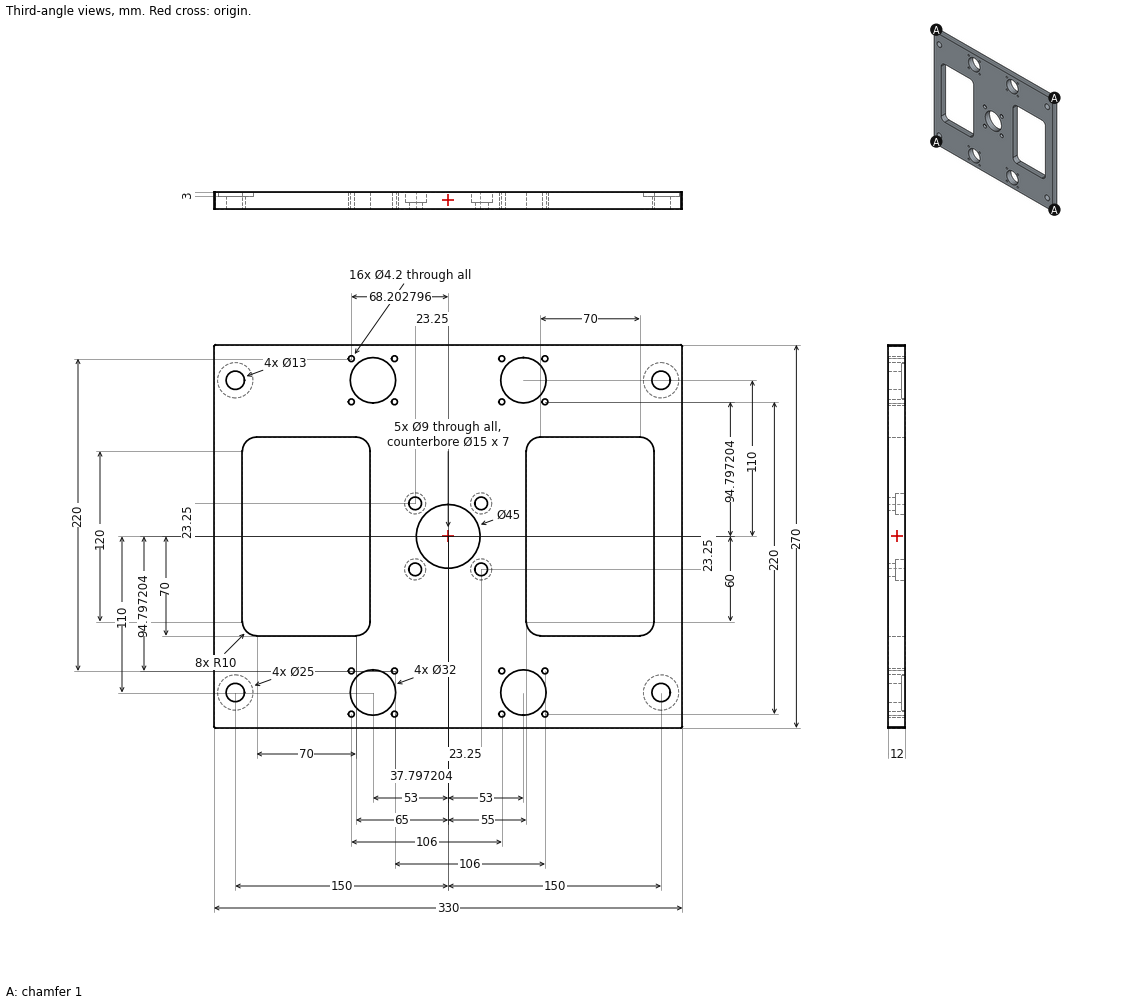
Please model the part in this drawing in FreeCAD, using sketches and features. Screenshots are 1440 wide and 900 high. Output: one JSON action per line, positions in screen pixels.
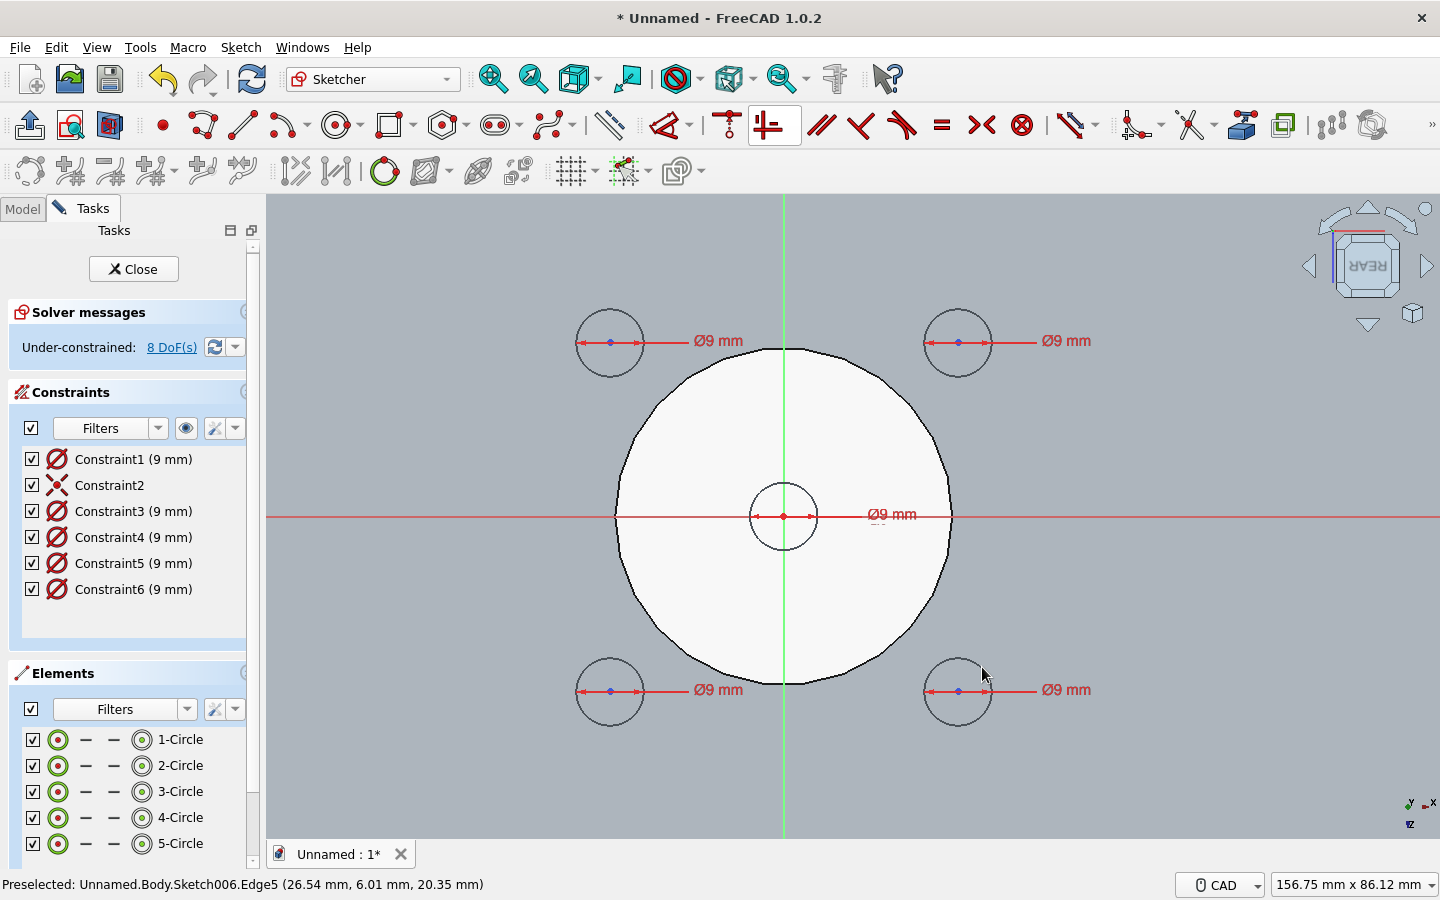
{"action": "left_click", "coordinate": [610, 692]}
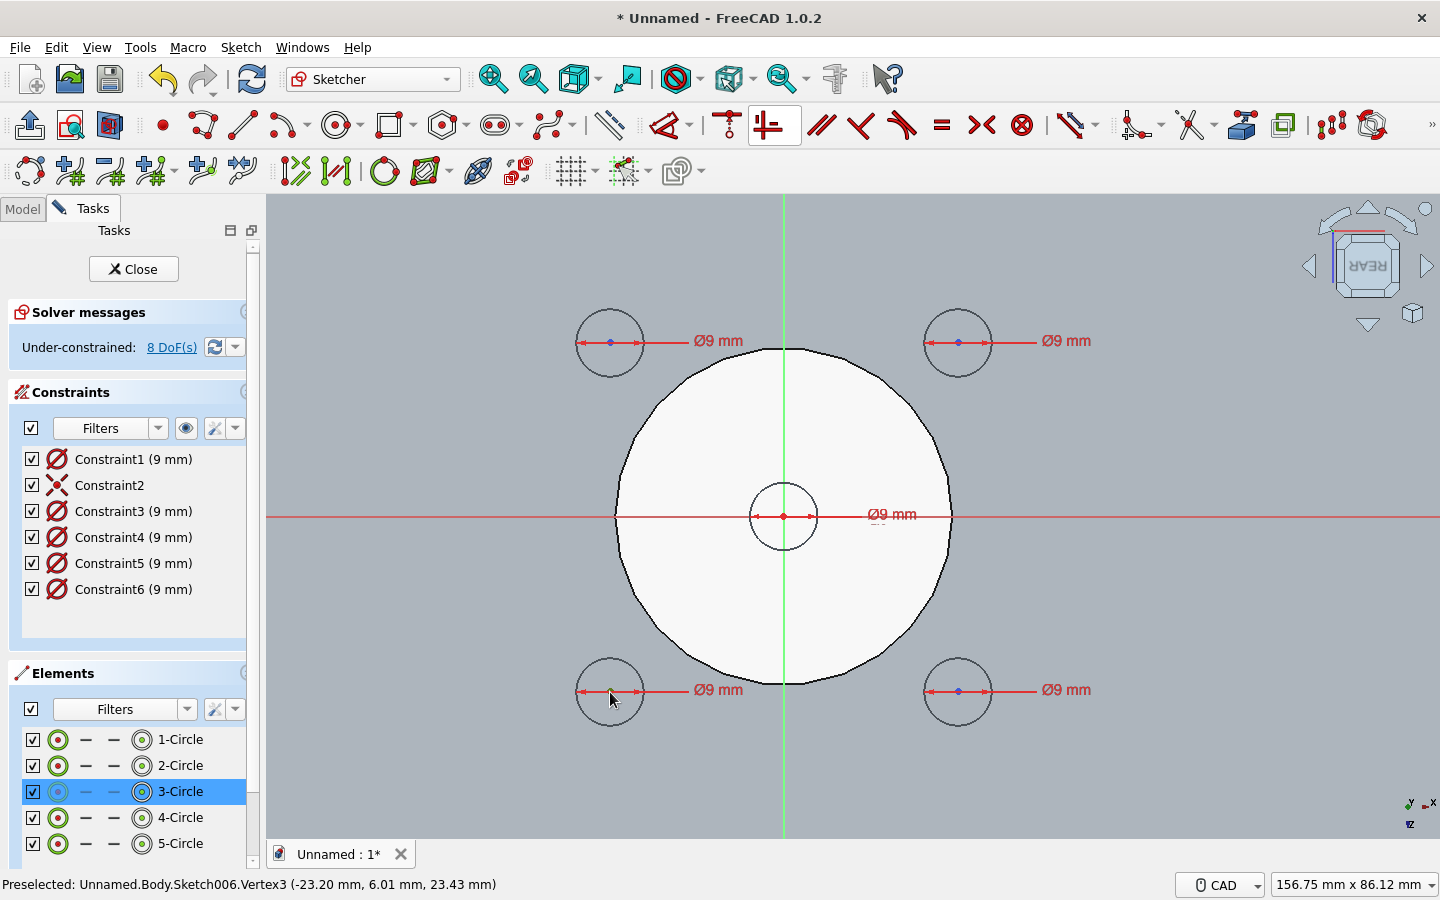
{"action": "left_click", "coordinate": [610, 343]}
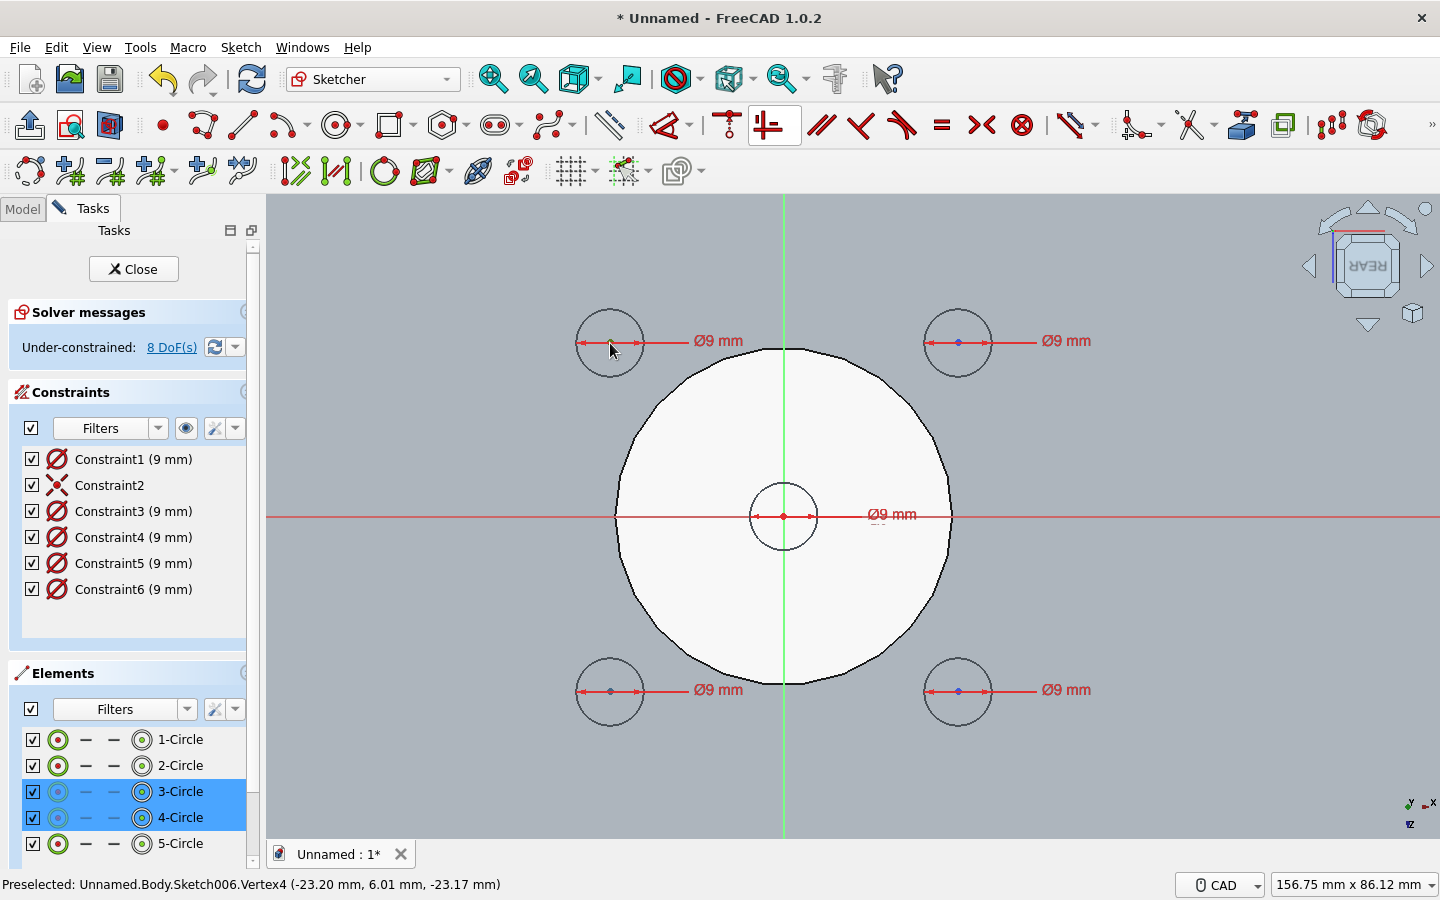
{"action": "key", "text": "v"}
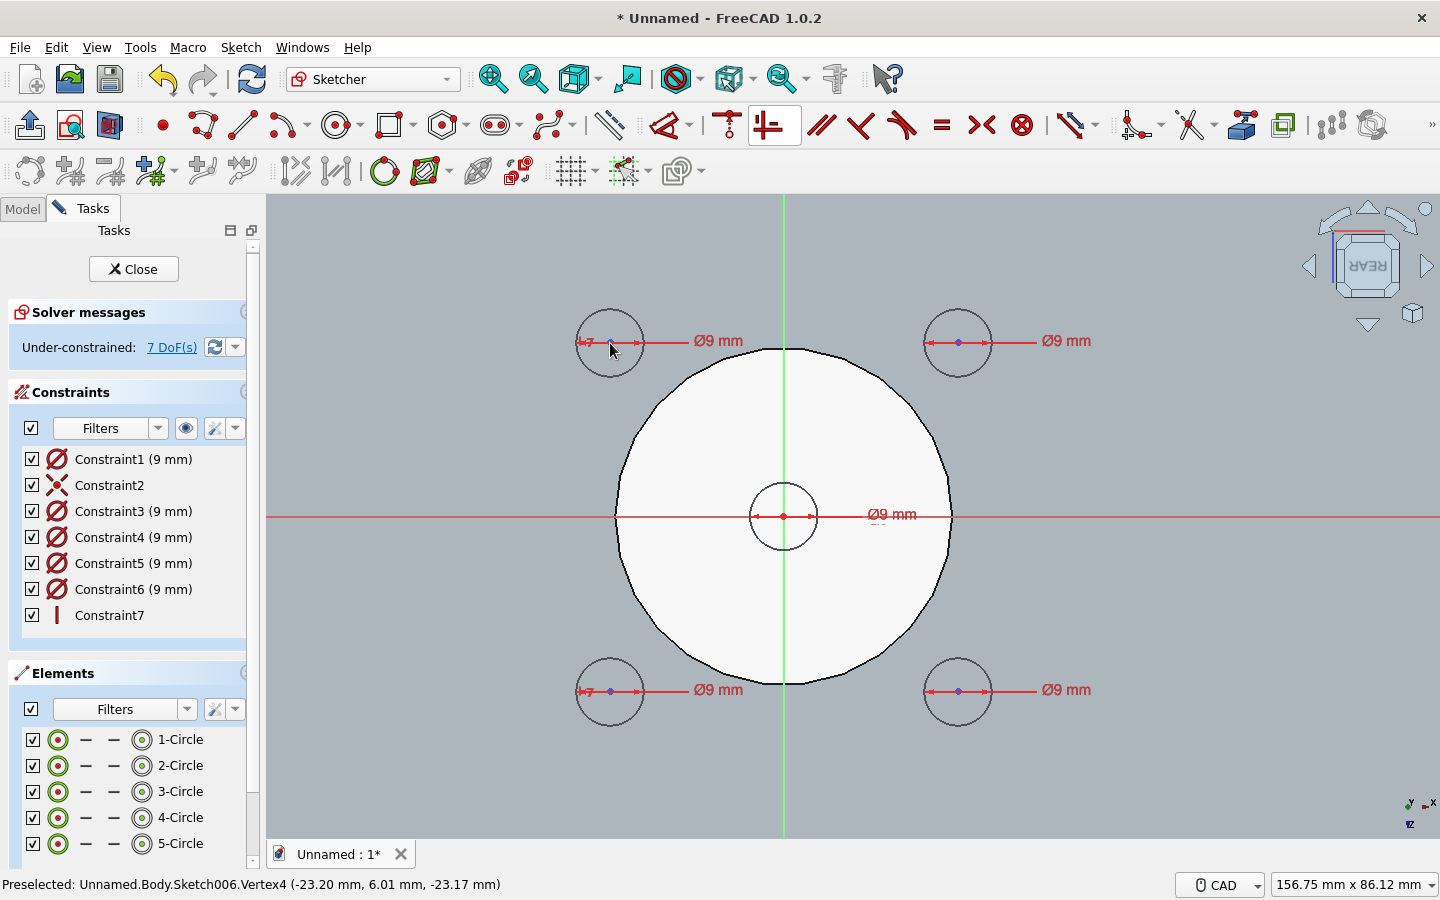
{"action": "left_click", "coordinate": [958, 343]}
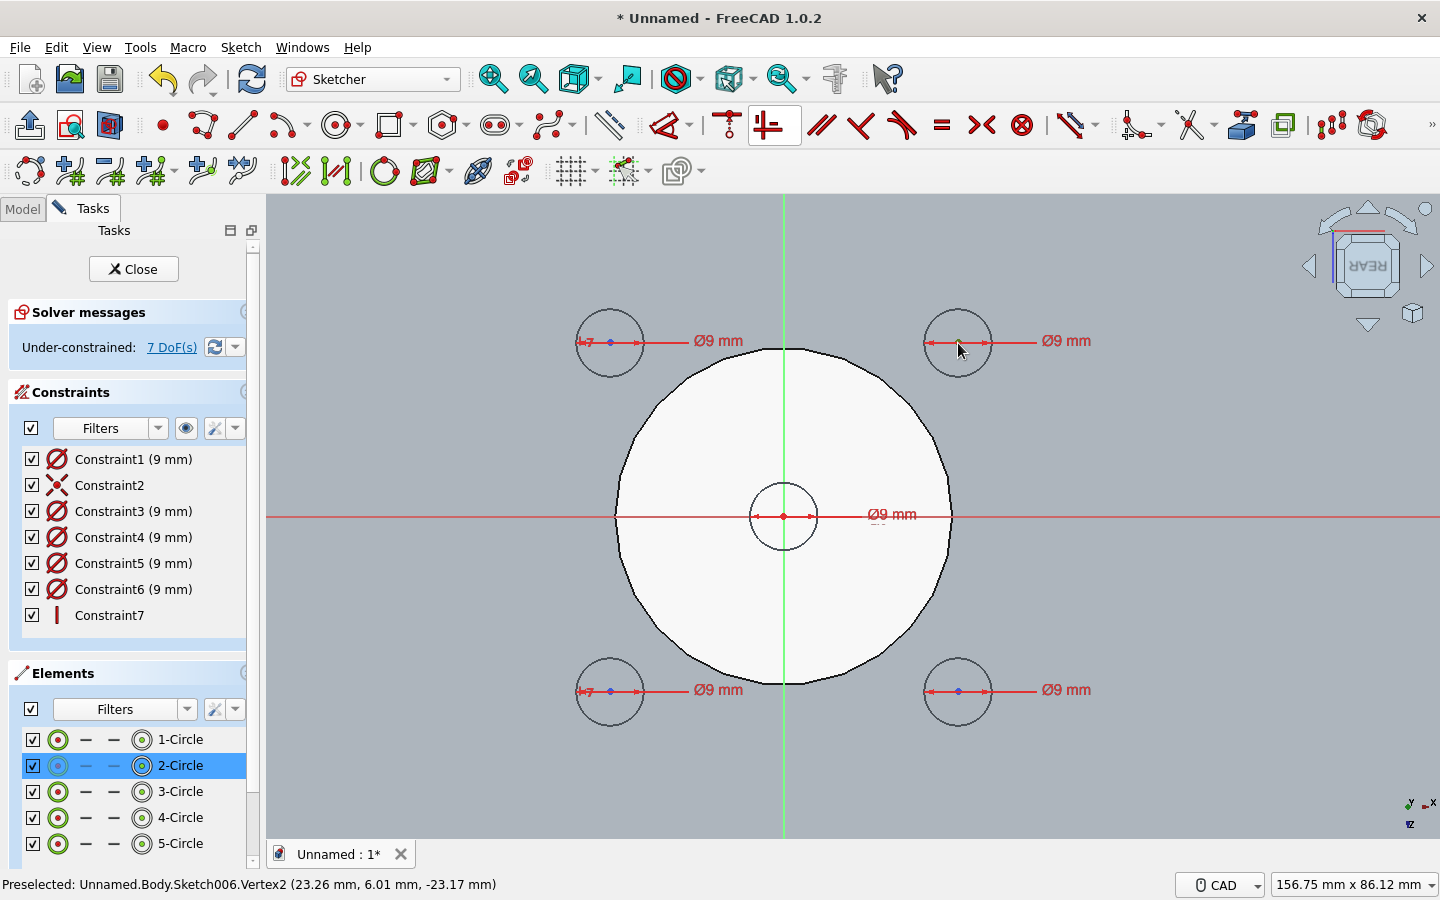
{"action": "left_click", "coordinate": [610, 343]}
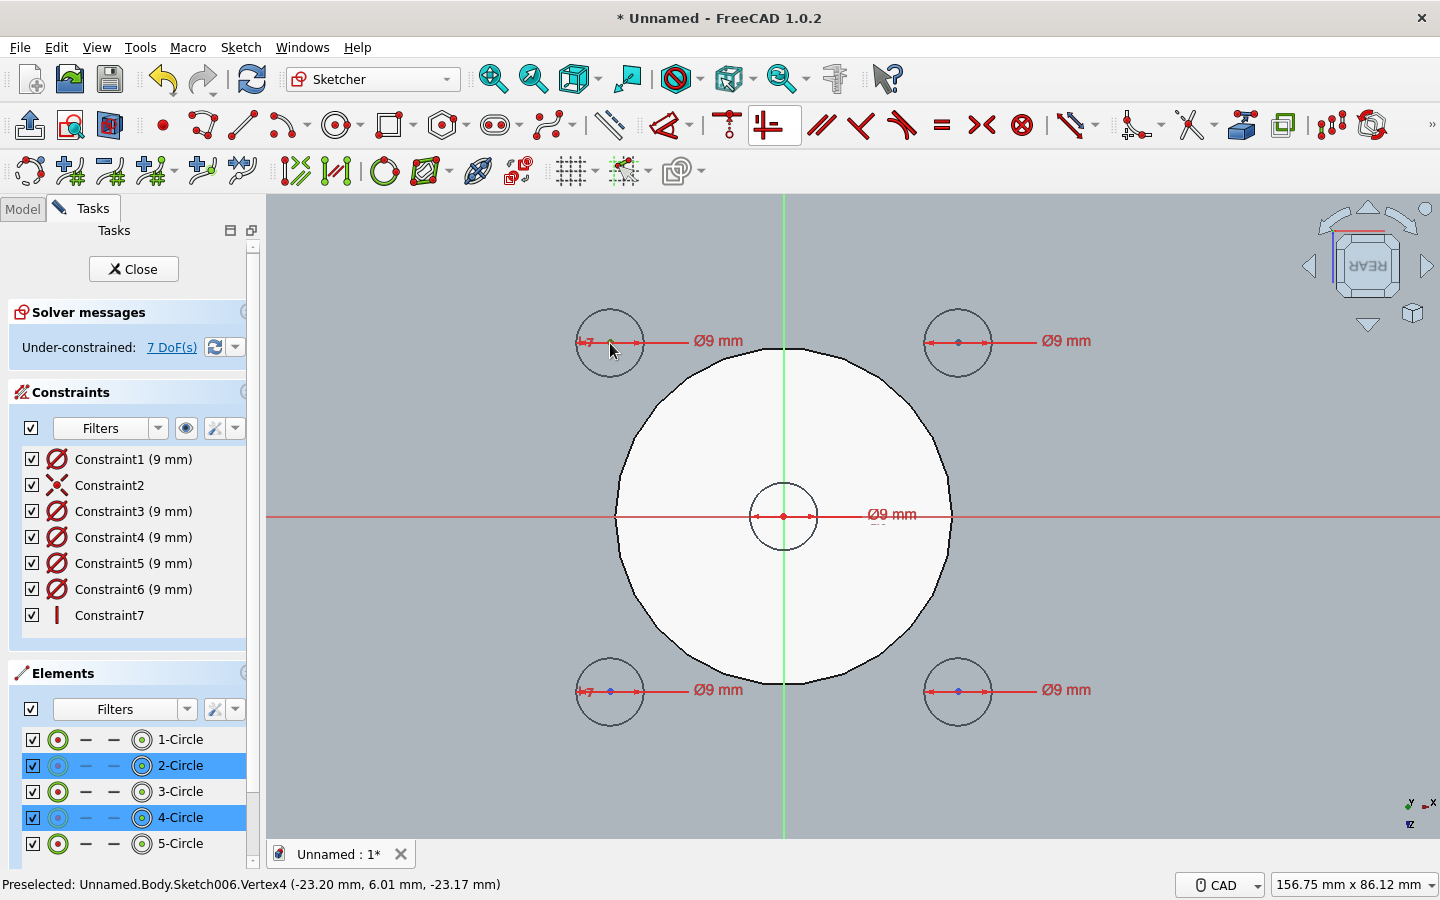
{"action": "left_click", "coordinate": [796, 126]}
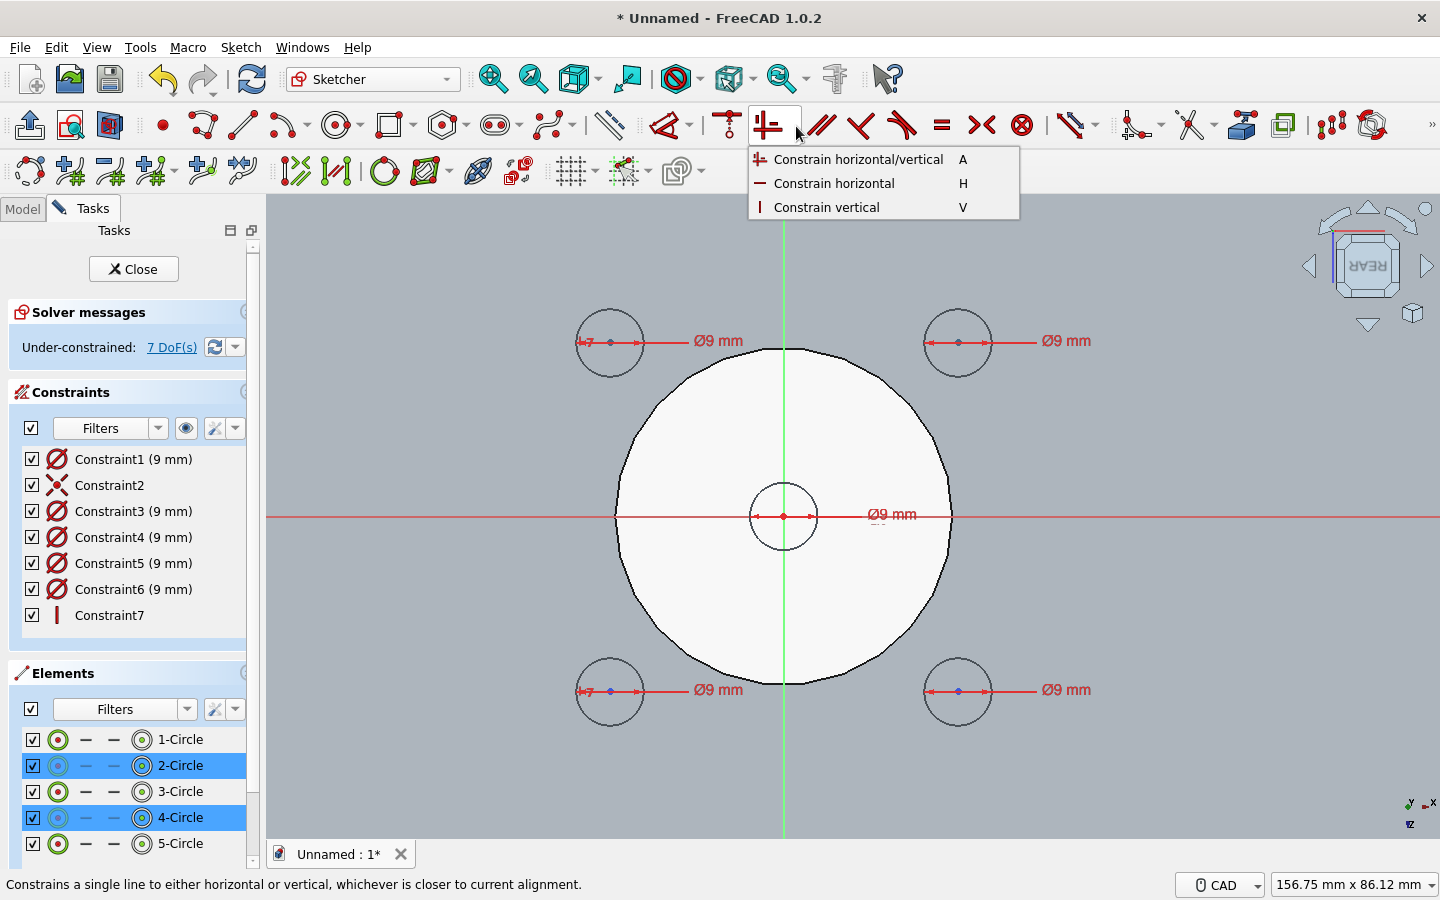
{"action": "left_click", "coordinate": [884, 183]}